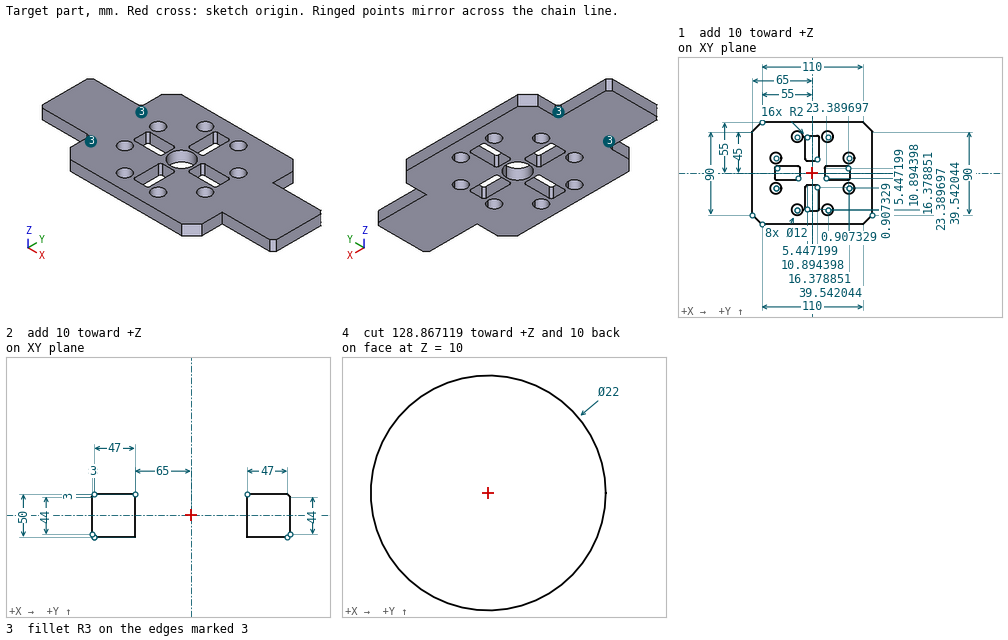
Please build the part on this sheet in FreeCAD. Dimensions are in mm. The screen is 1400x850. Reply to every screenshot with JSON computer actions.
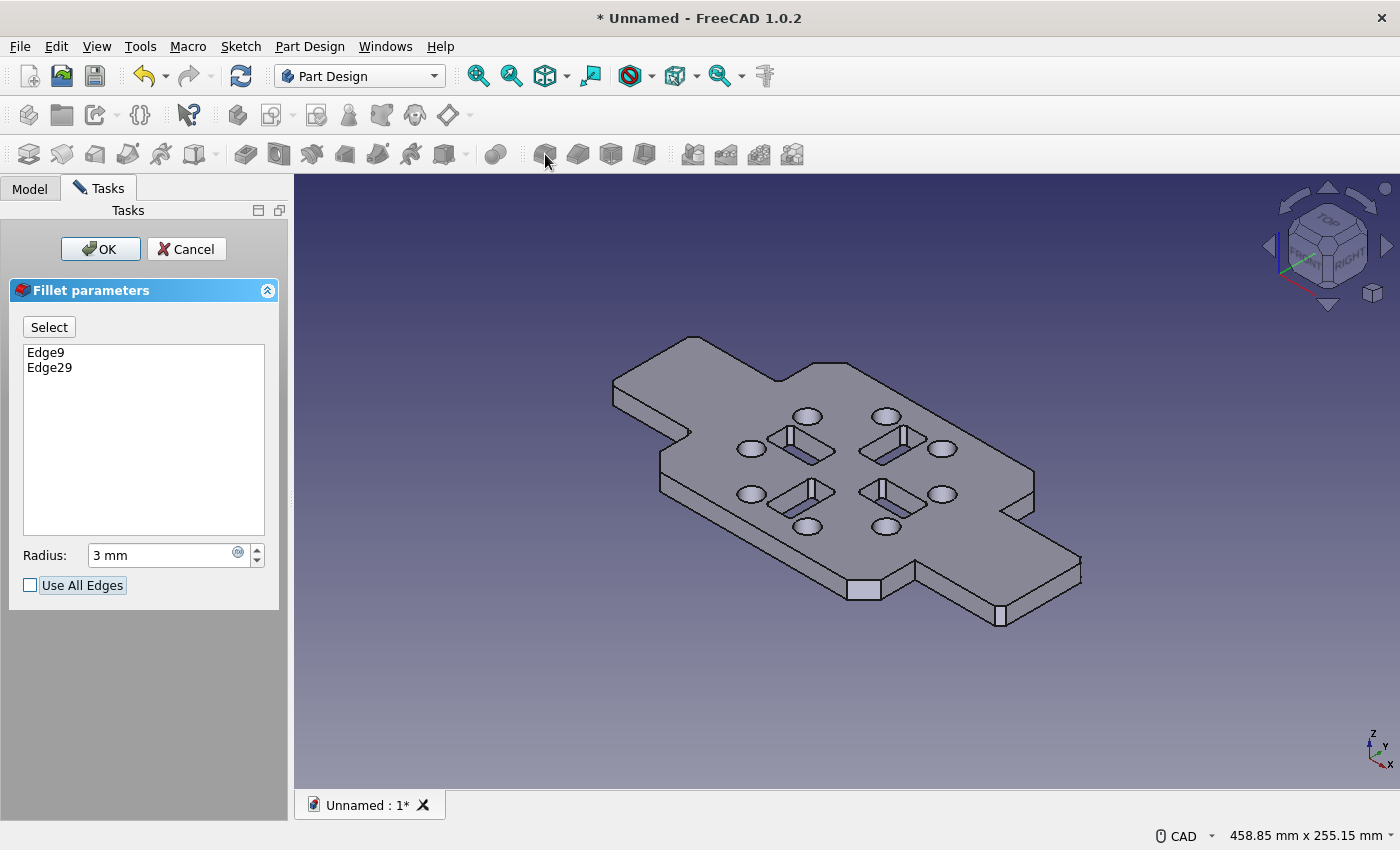
{"action": "left_click", "coordinate": [101, 249]}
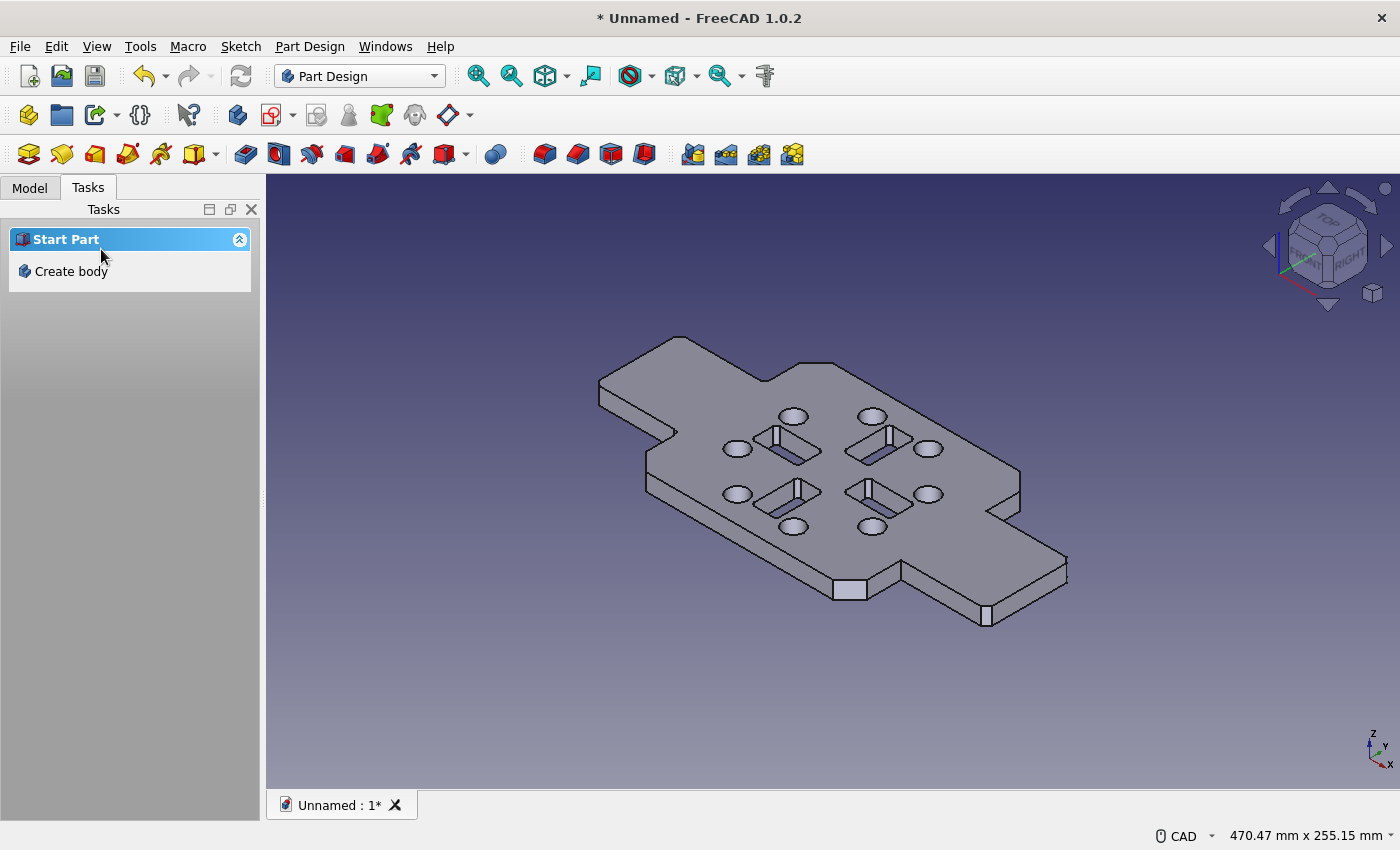
{"action": "left_click", "coordinate": [721, 406]}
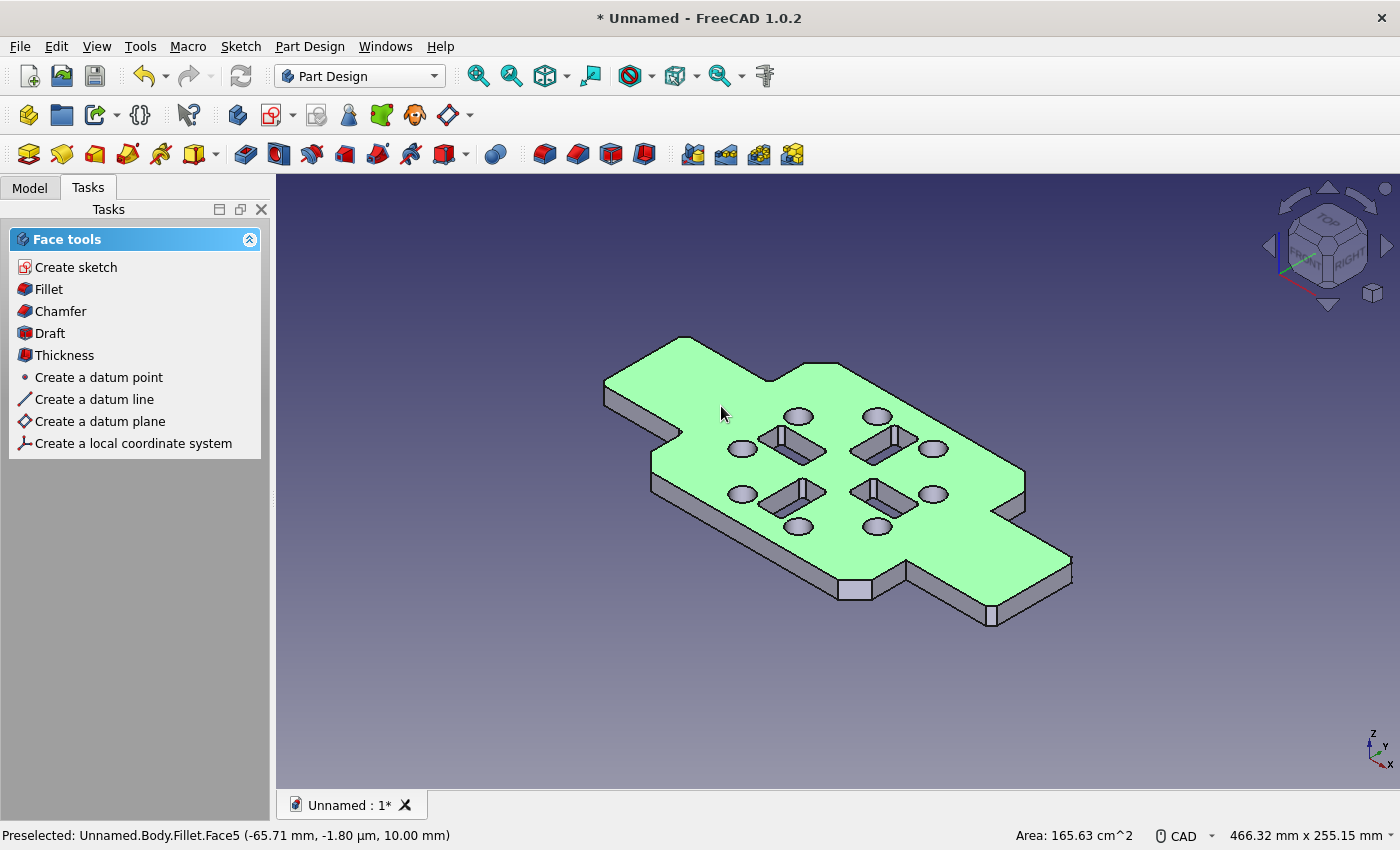
{"action": "left_click", "coordinate": [270, 116]}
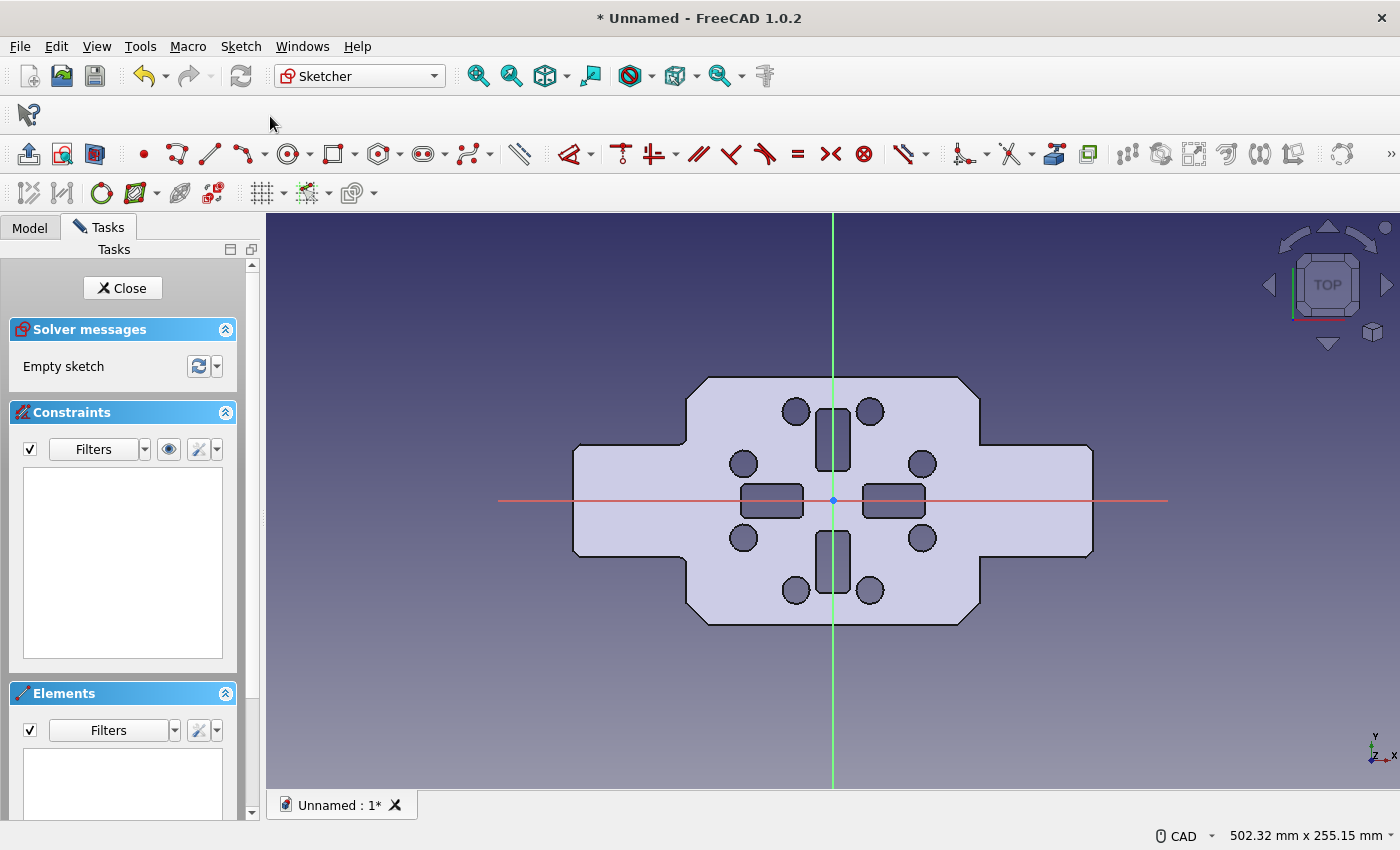
{"action": "scroll", "coordinate": [844, 501], "scroll_direction": "up", "scroll_amount": 10}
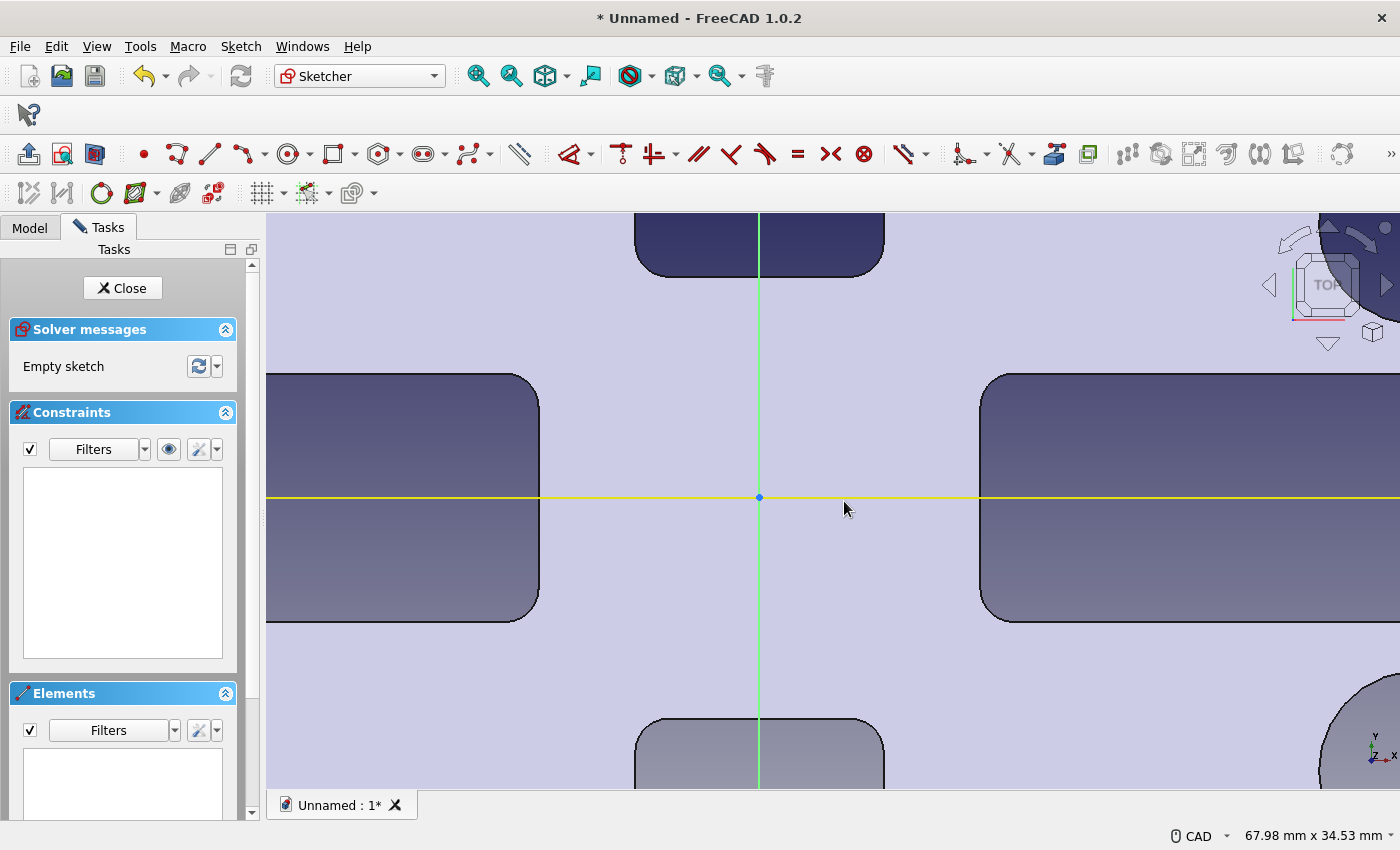
{"action": "left_click", "coordinate": [288, 154]}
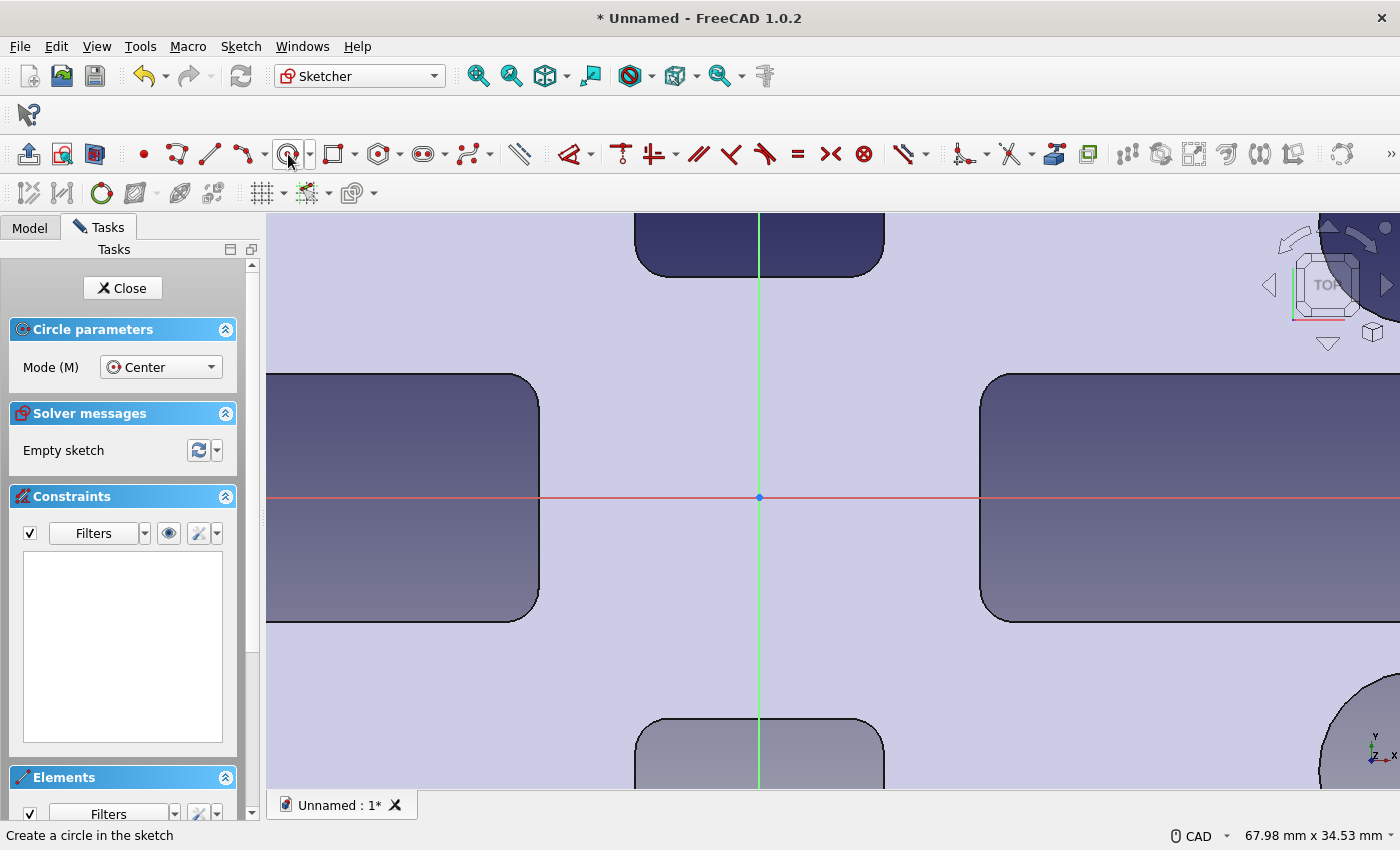
{"action": "left_click", "coordinate": [759, 498]}
{"action": "mouse_move", "coordinate": [889, 368]}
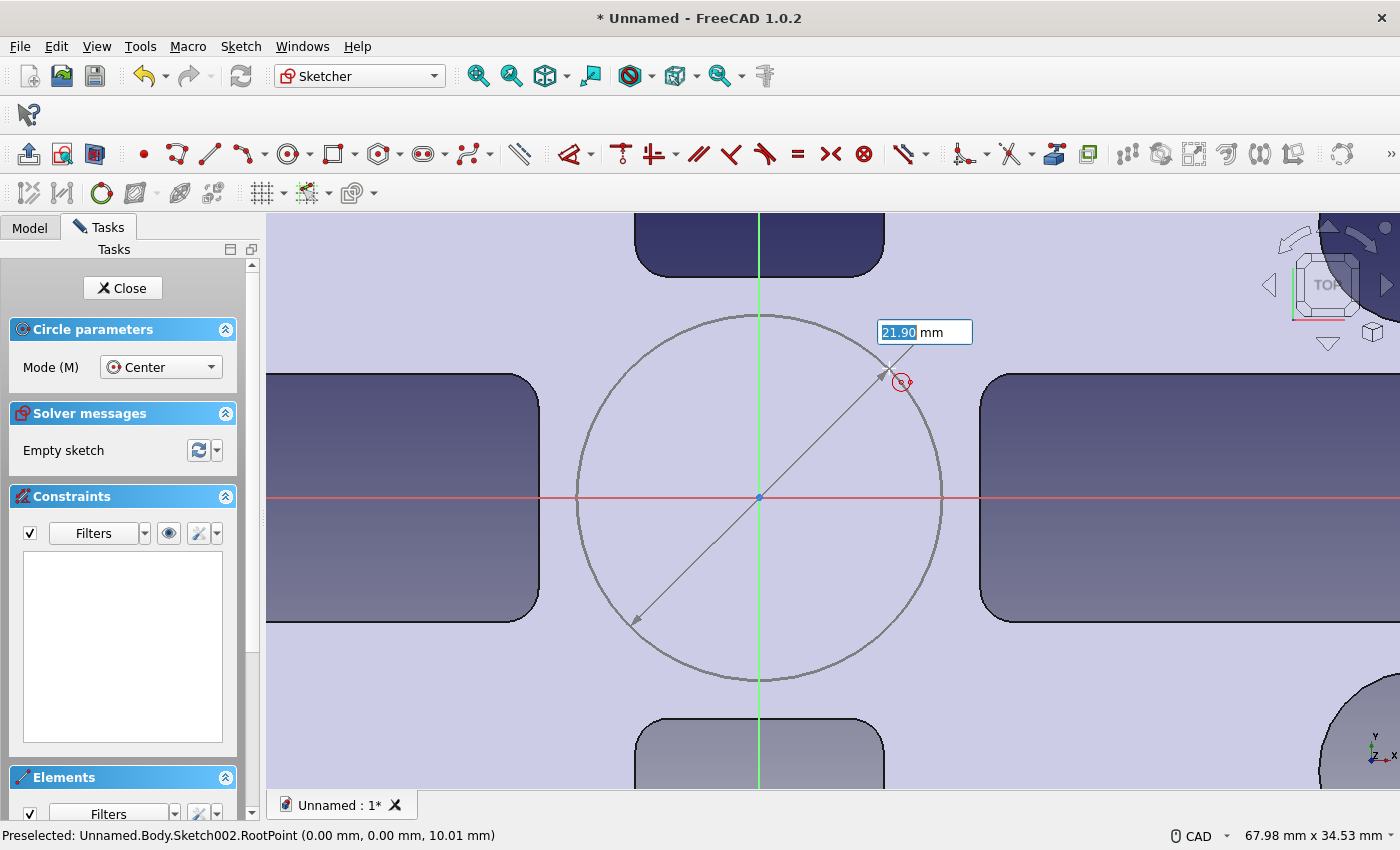
{"action": "type", "text": "22"}
{"action": "key", "text": "Return"}
{"action": "key", "text": "Escape"}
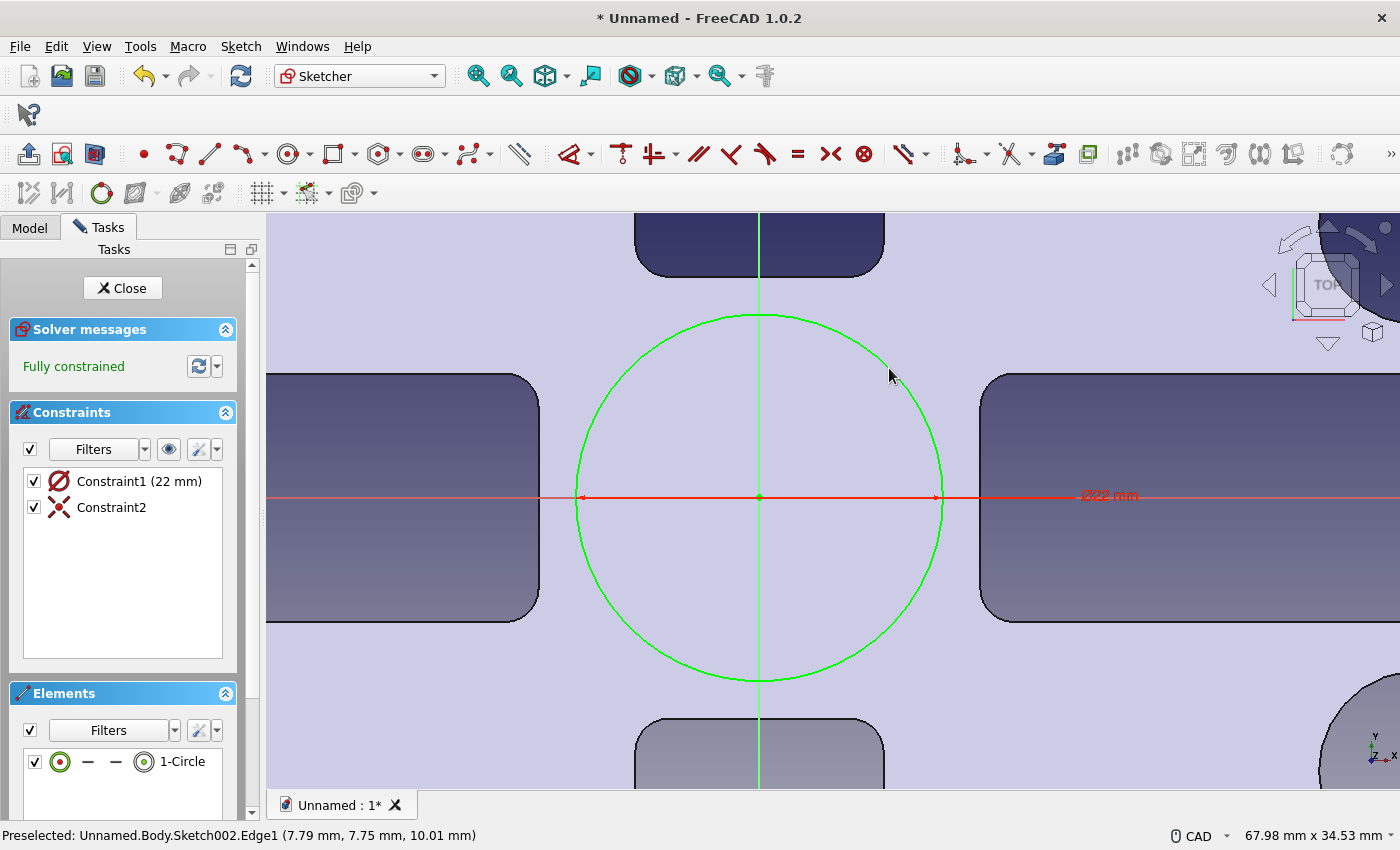
{"action": "left_click", "coordinate": [123, 288]}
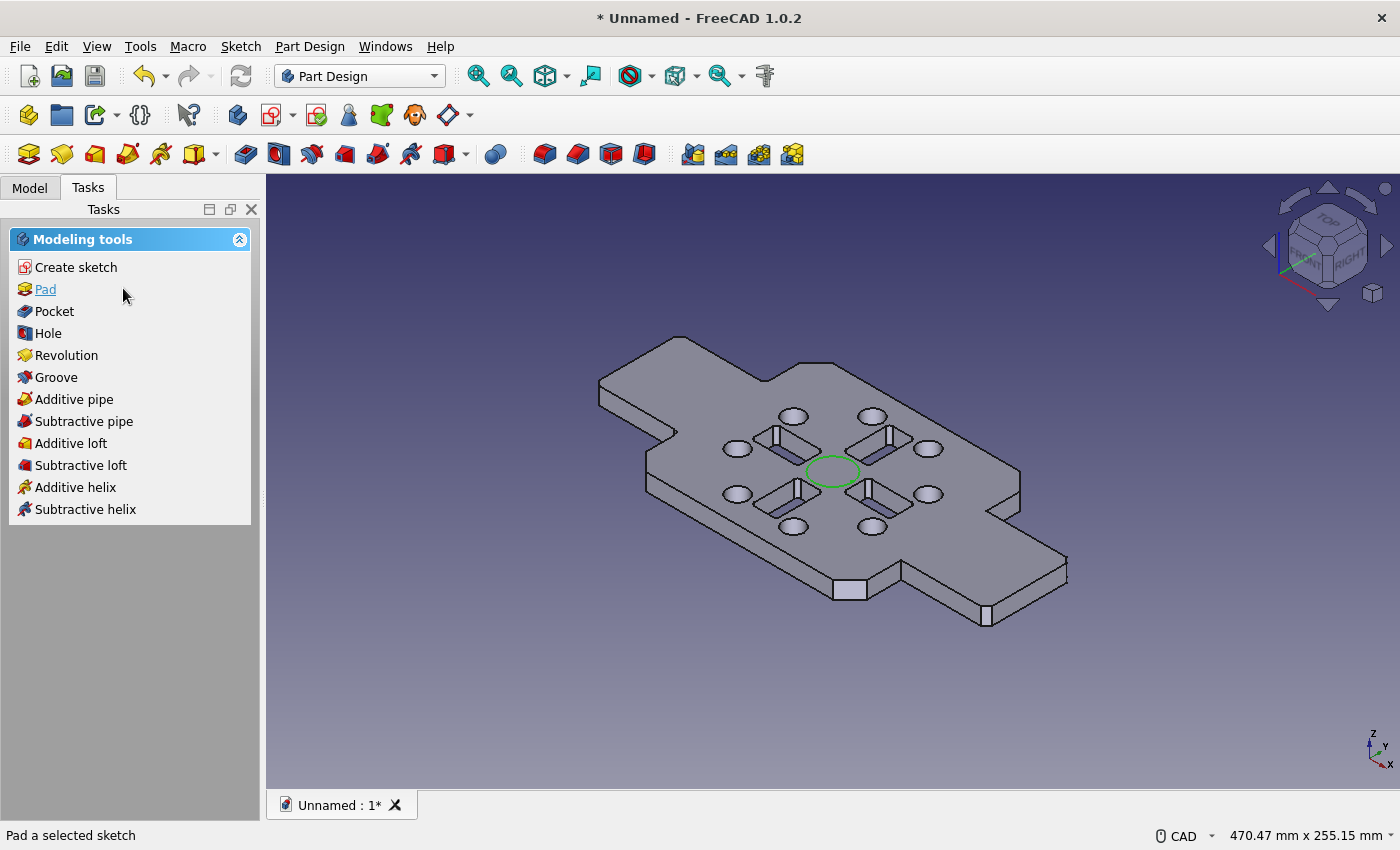
{"action": "left_click", "coordinate": [246, 154]}